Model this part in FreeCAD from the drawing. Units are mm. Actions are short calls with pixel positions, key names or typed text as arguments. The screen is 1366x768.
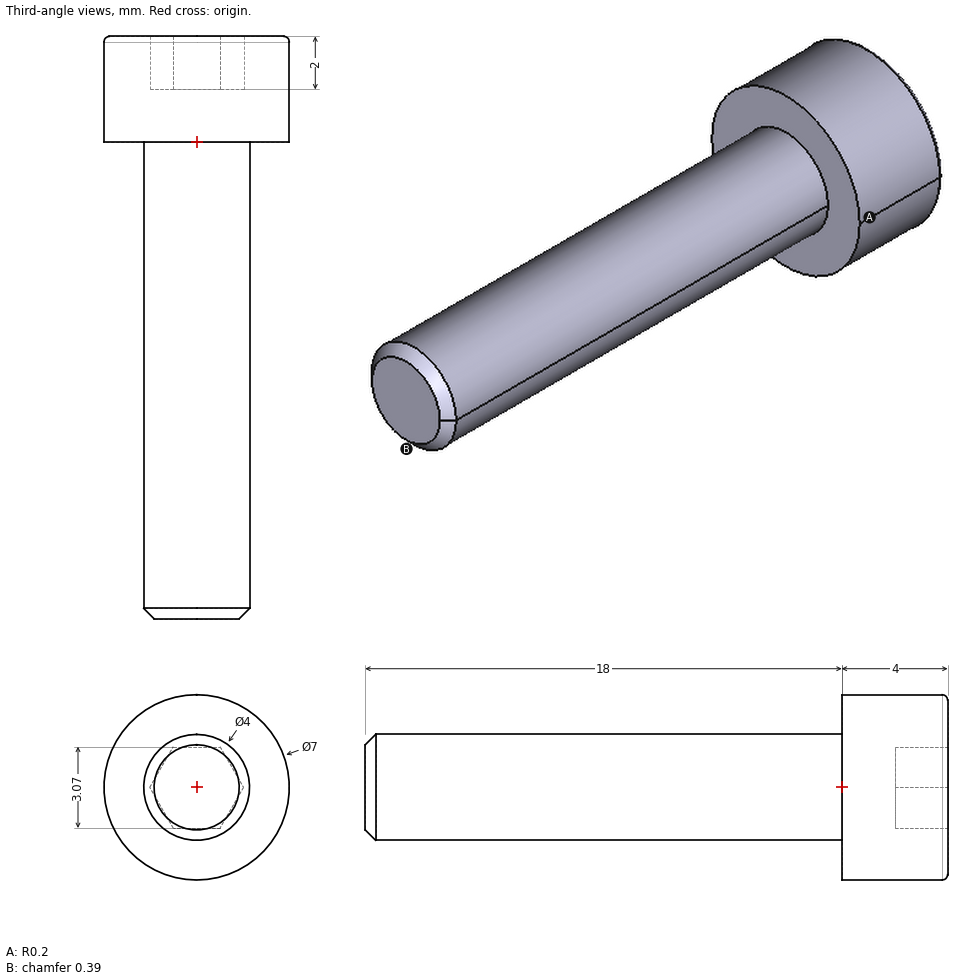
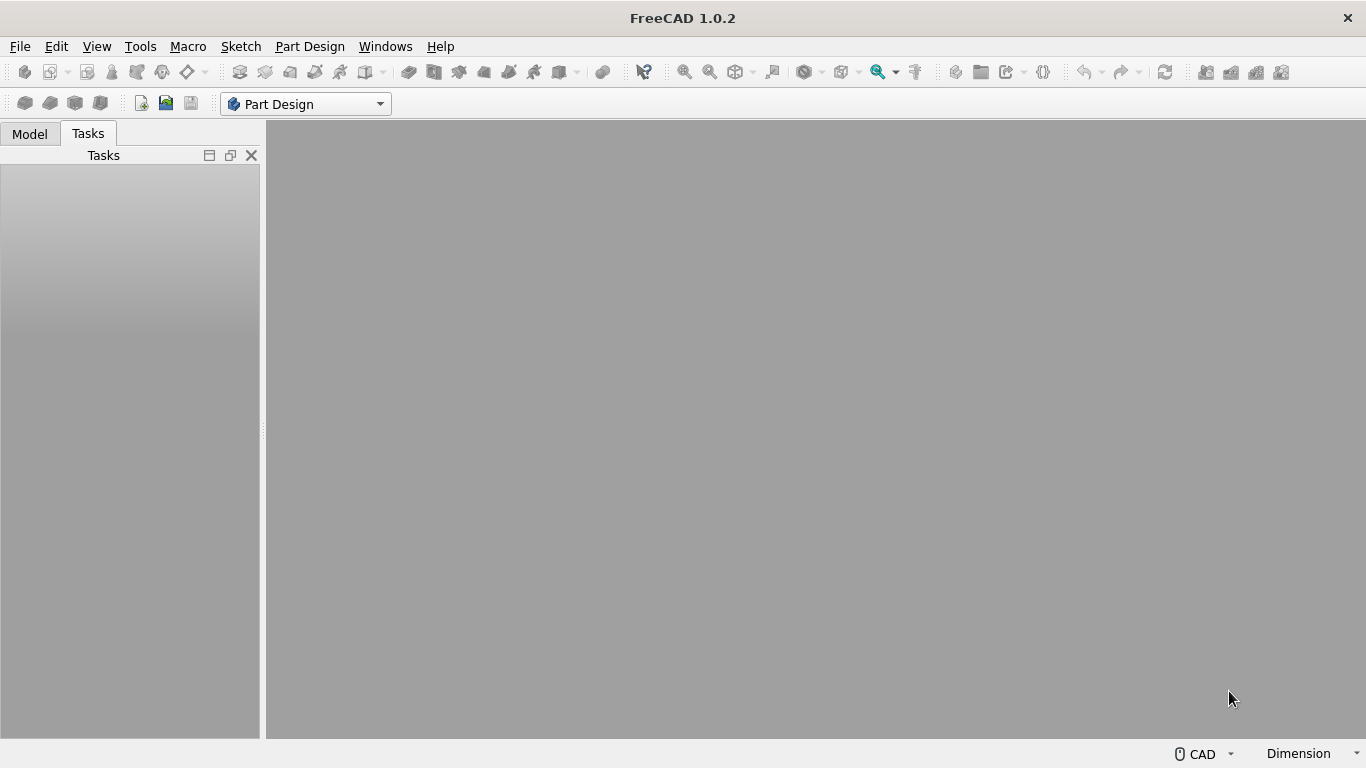
click(141, 104)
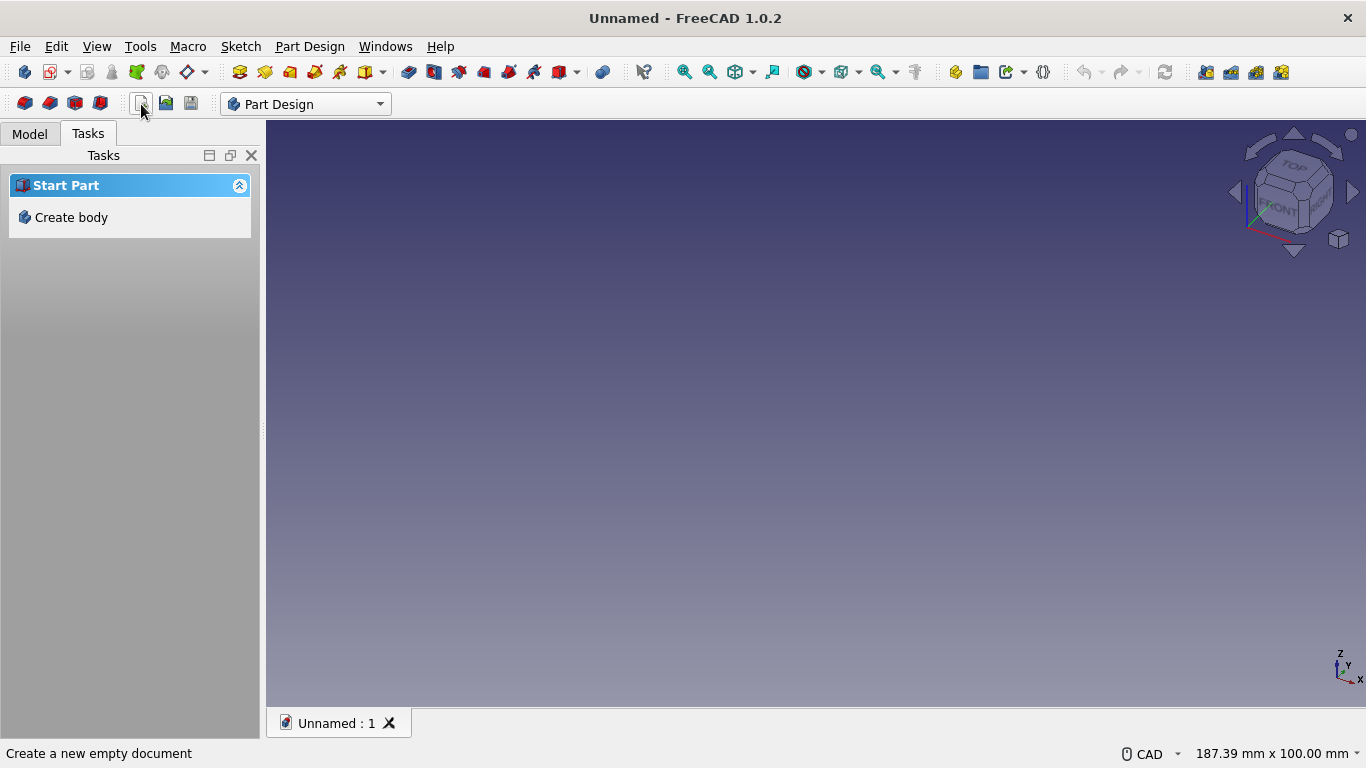
click(50, 72)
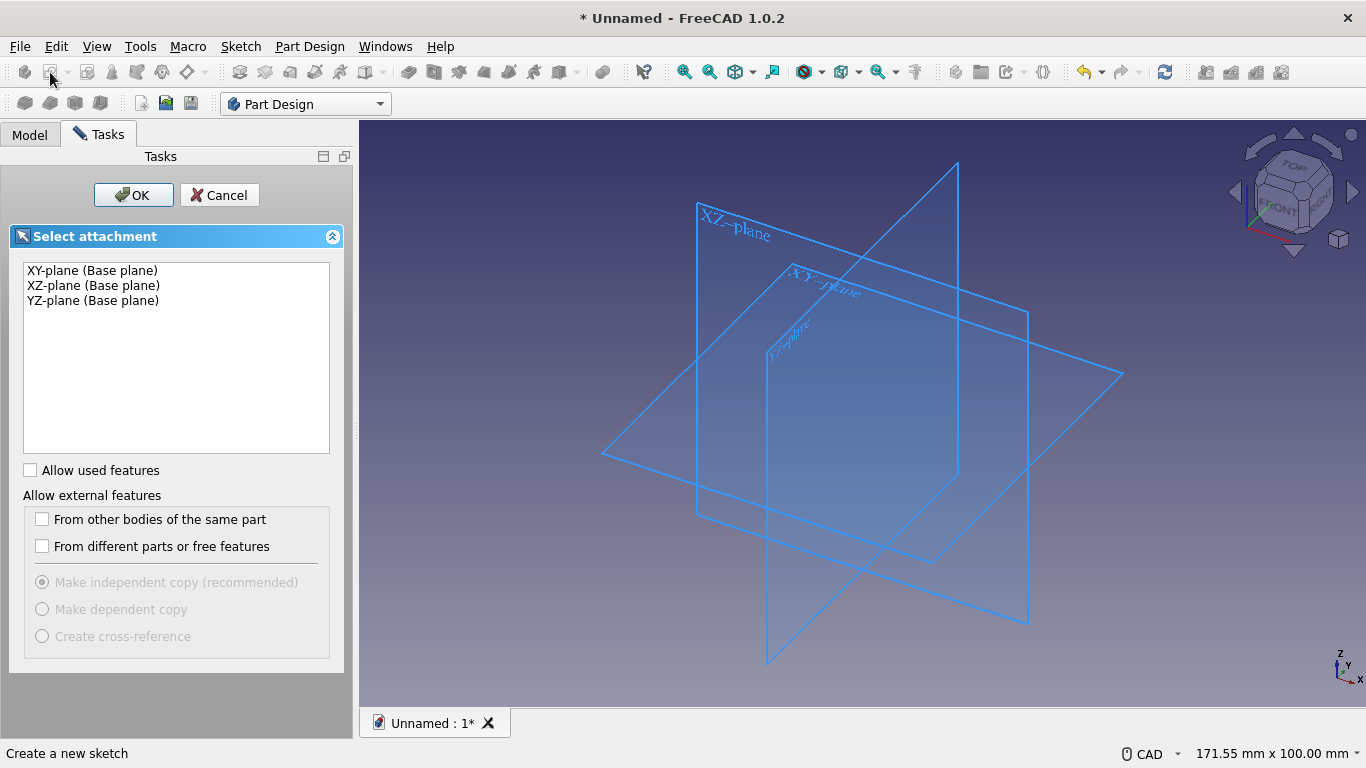
click(84, 286)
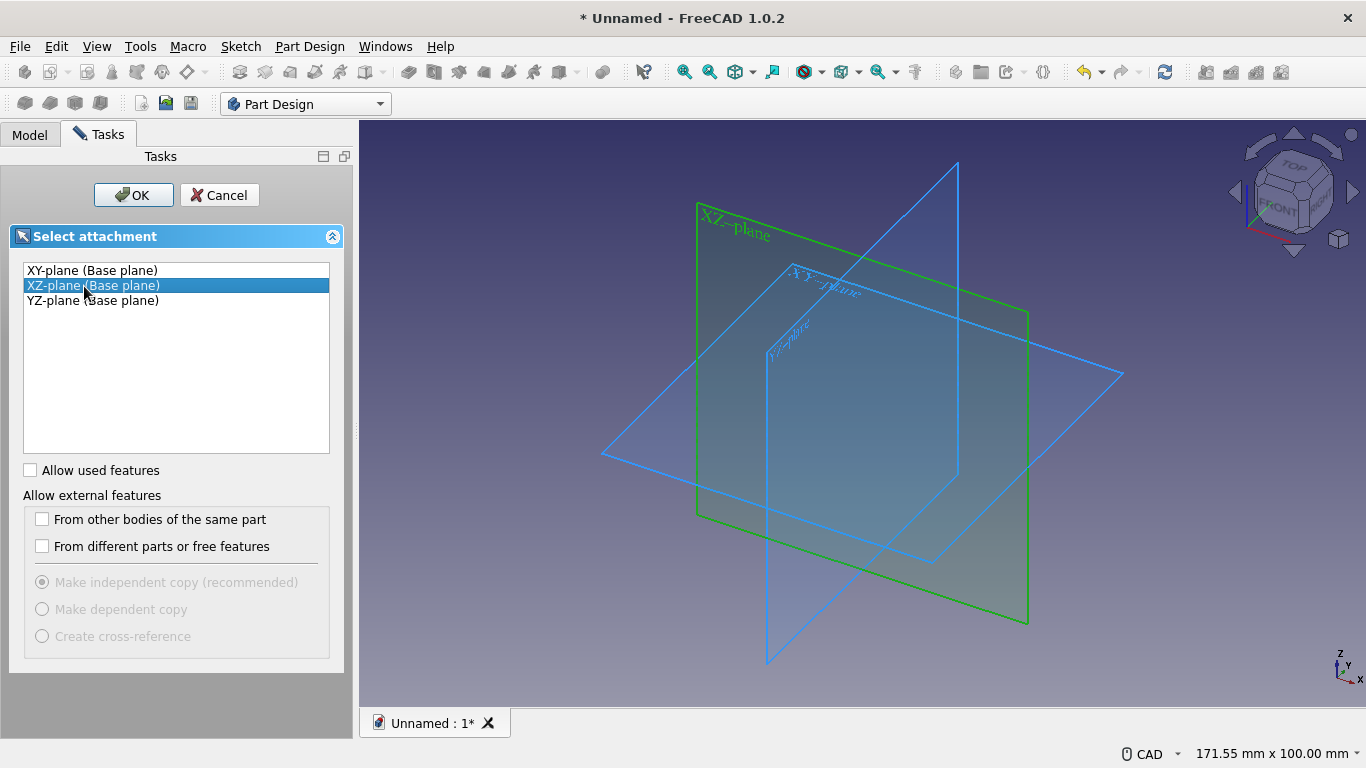
click(134, 195)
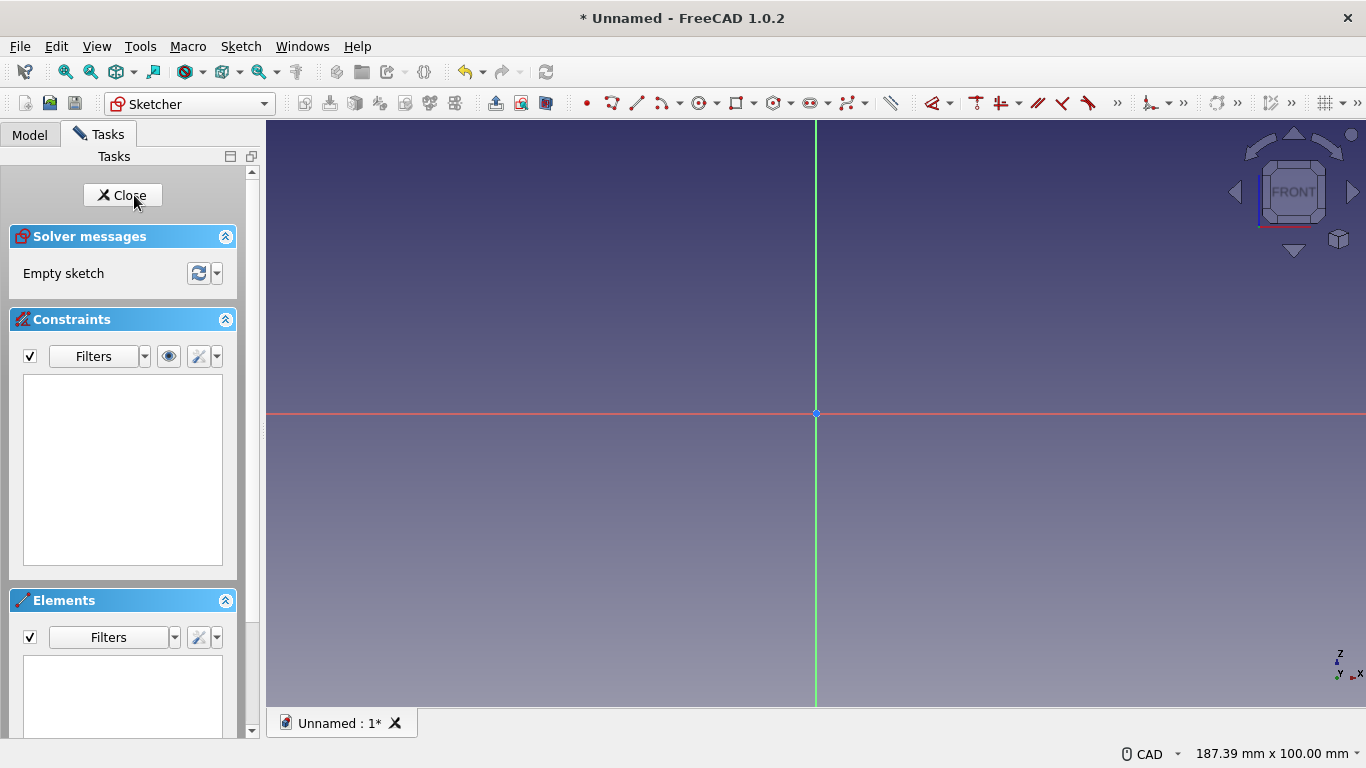
scroll(825, 414, up, 11)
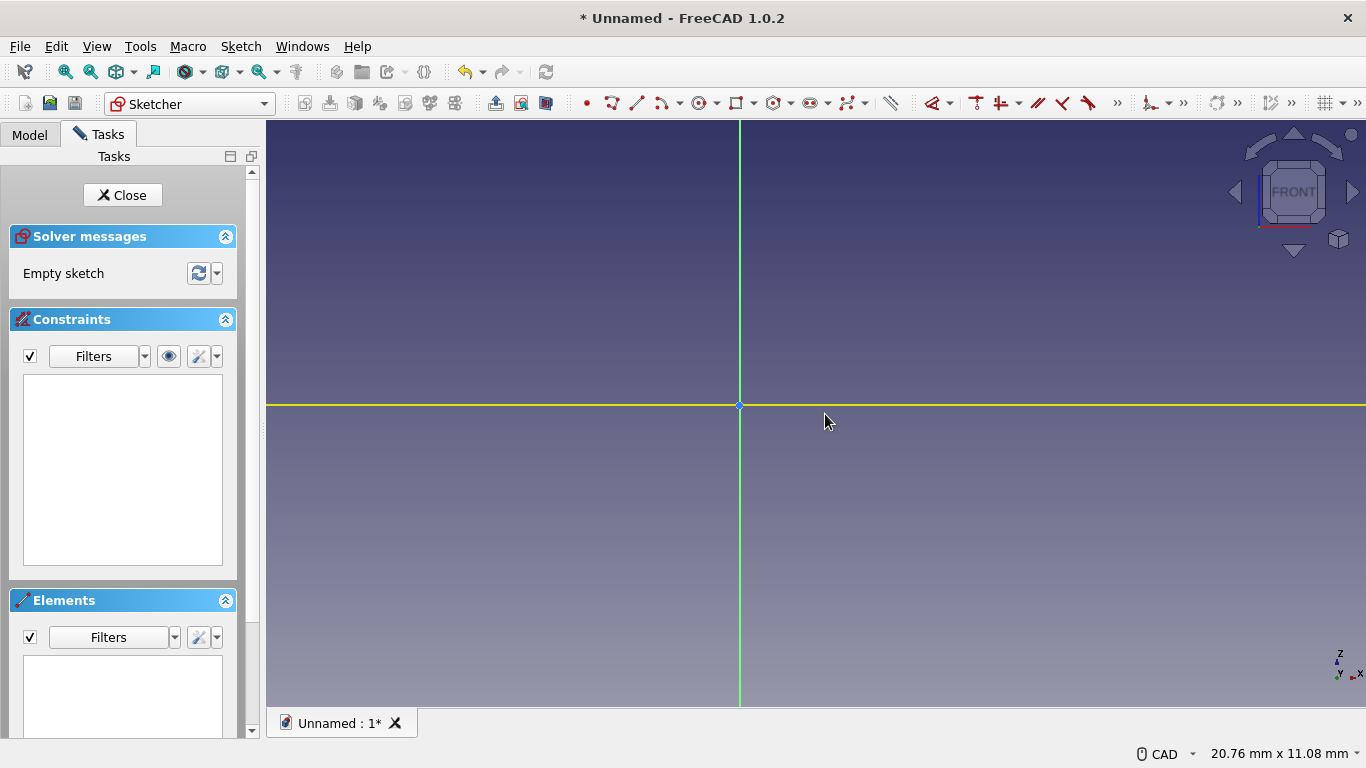
click(698, 104)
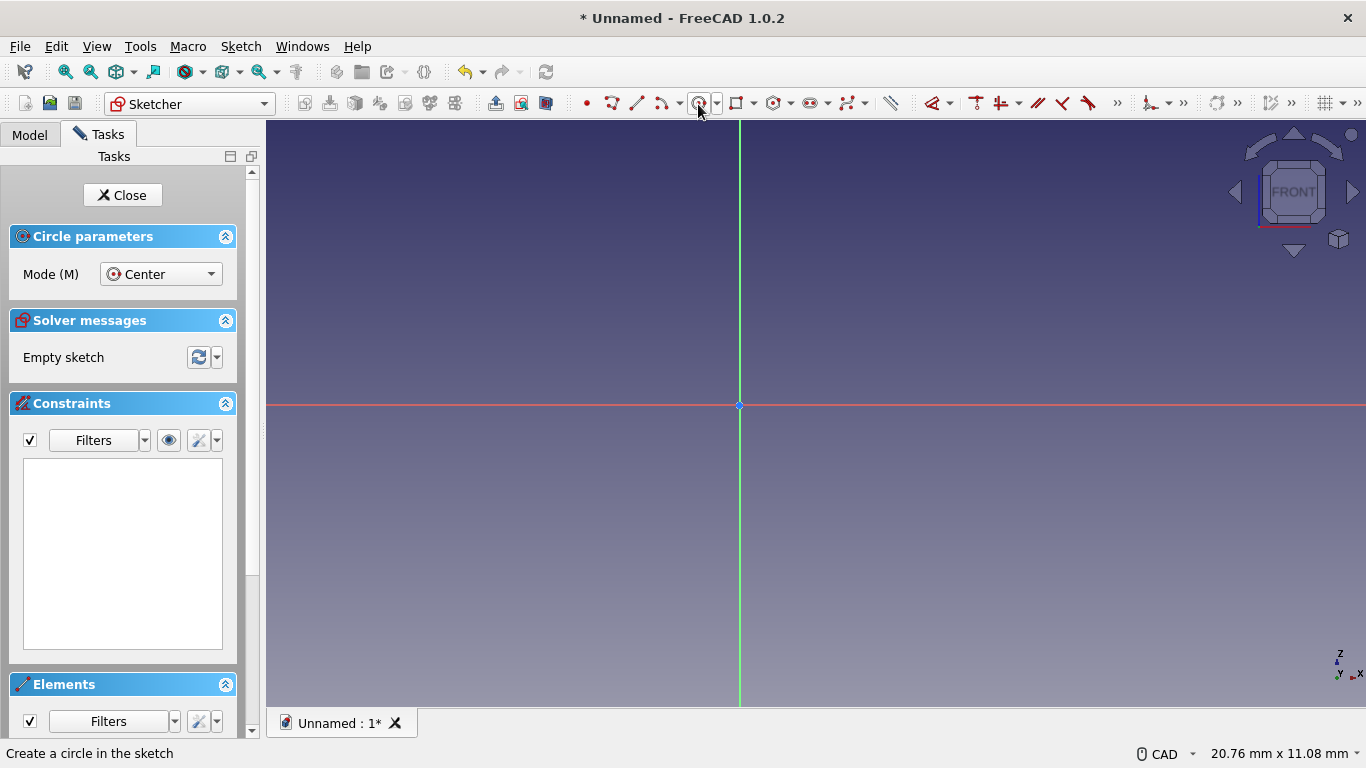
click(740, 405)
click(871, 274)
key(Escape)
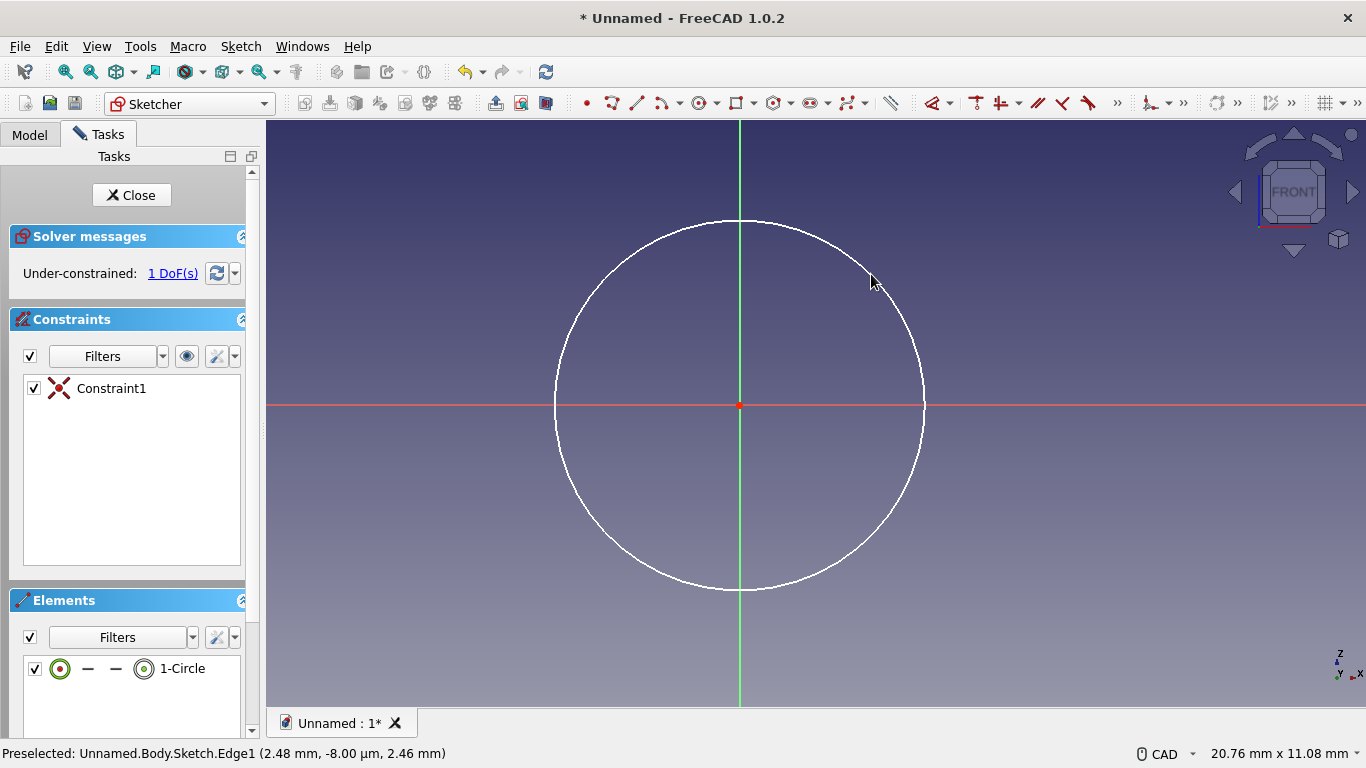
click(932, 104)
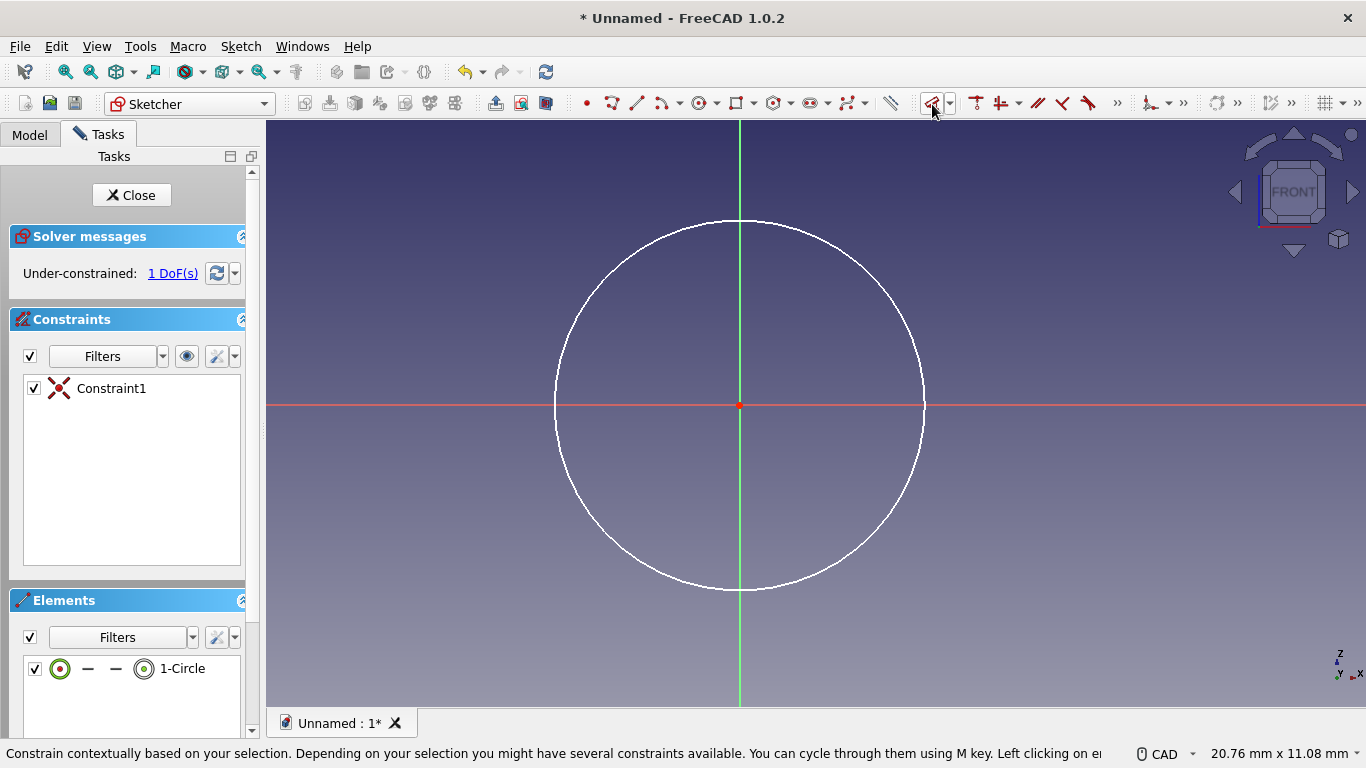
click(870, 274)
click(893, 251)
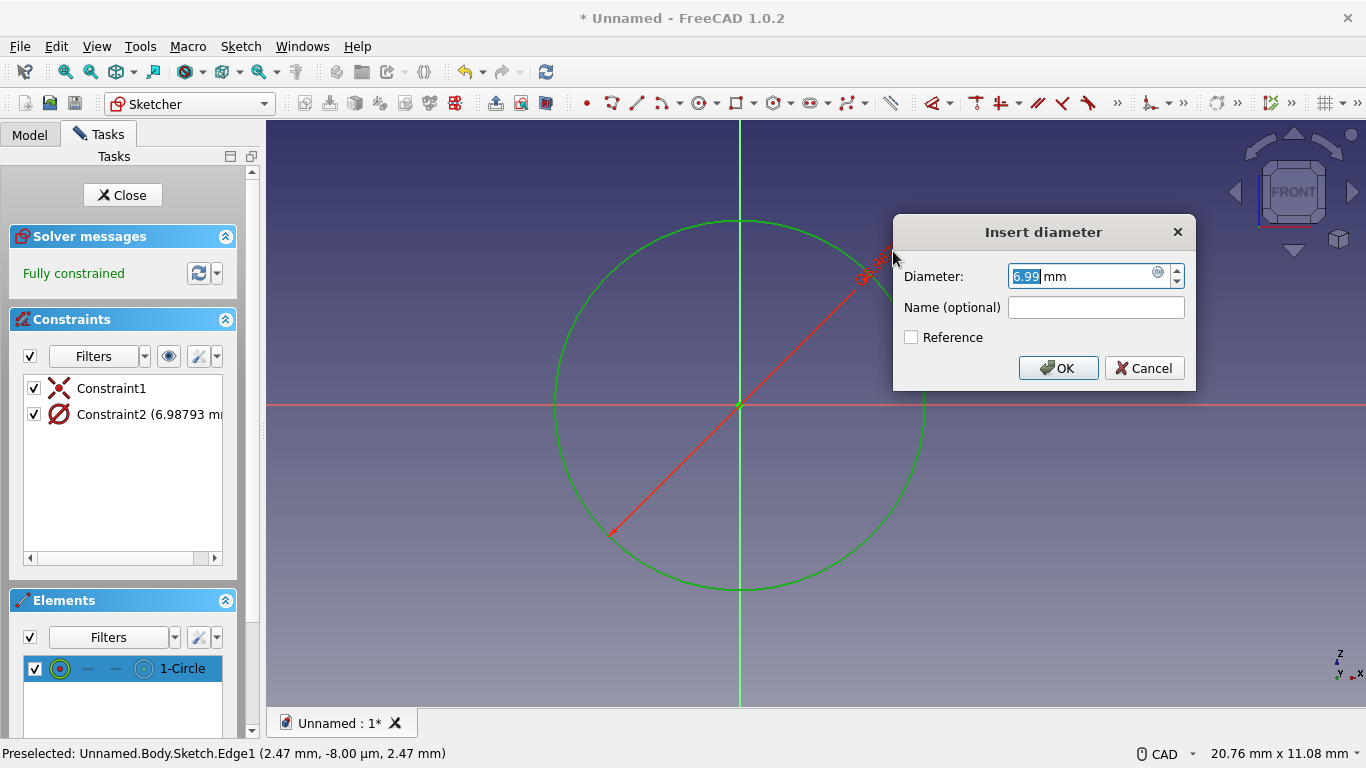
text(7)
key(Return)
key(Escape)